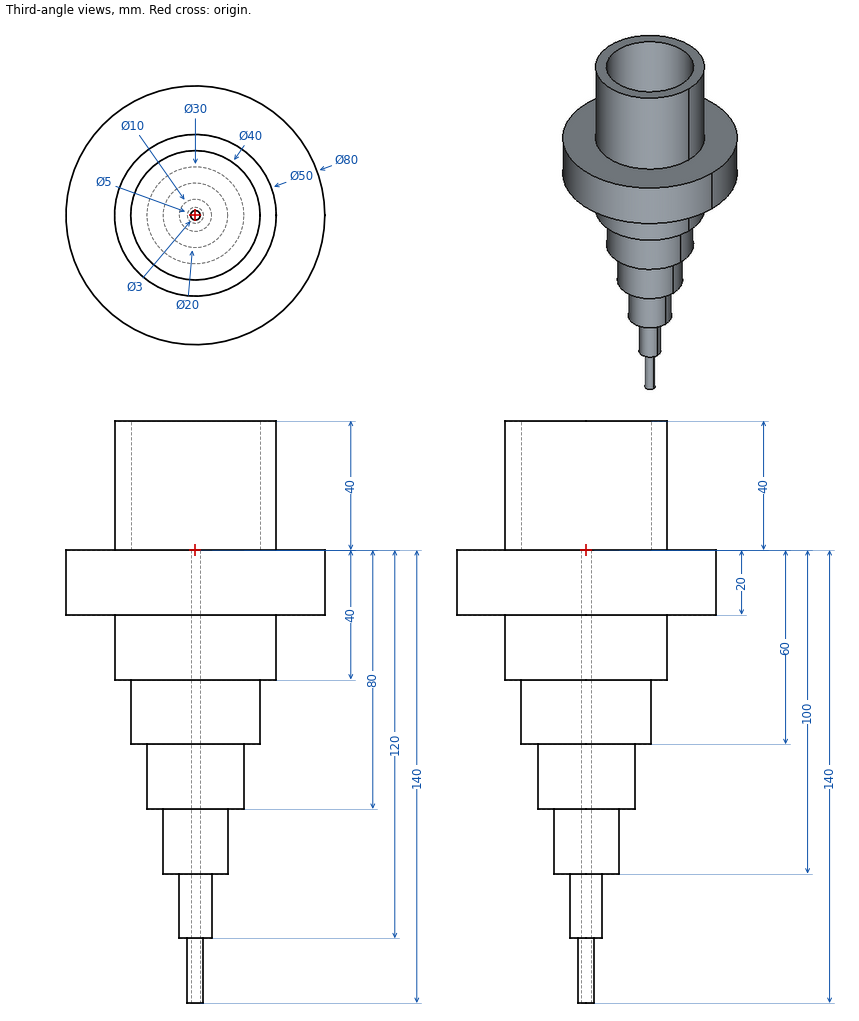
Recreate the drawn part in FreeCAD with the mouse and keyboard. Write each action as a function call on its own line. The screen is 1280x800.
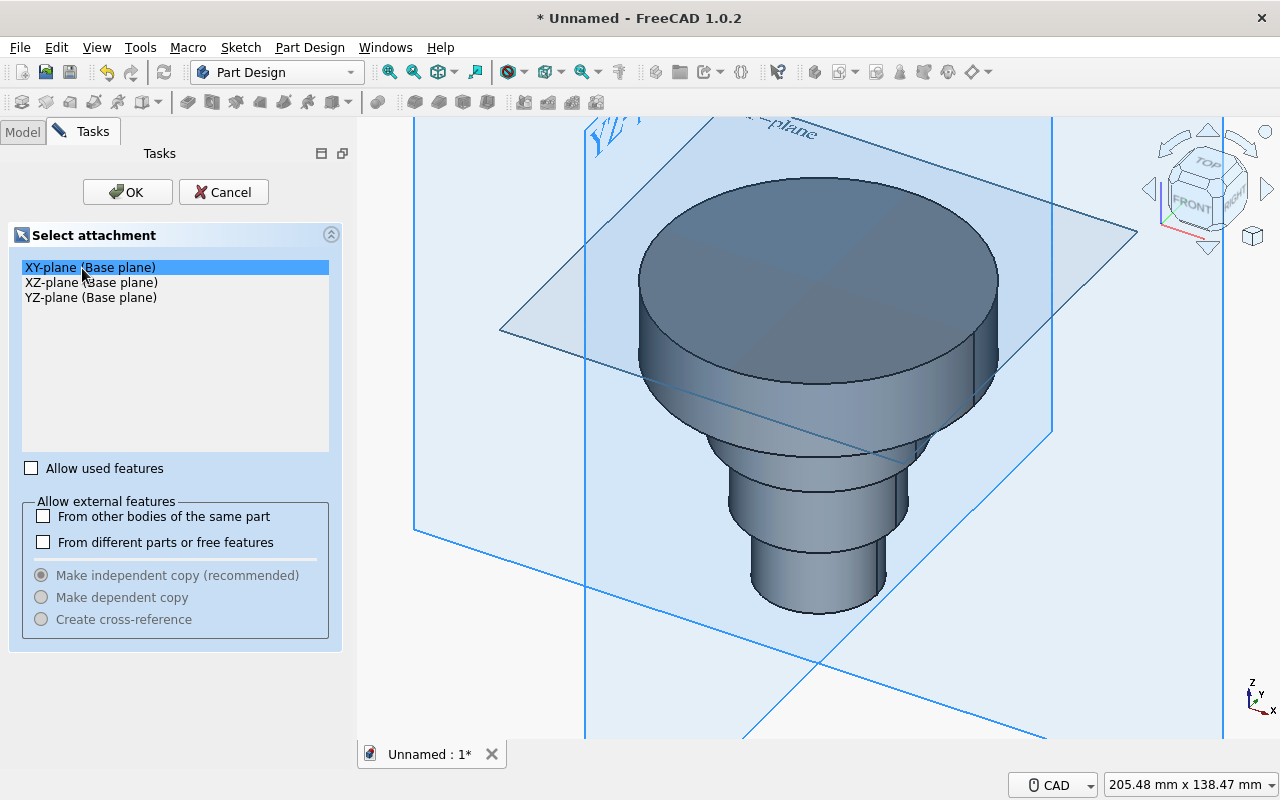
click(128, 192)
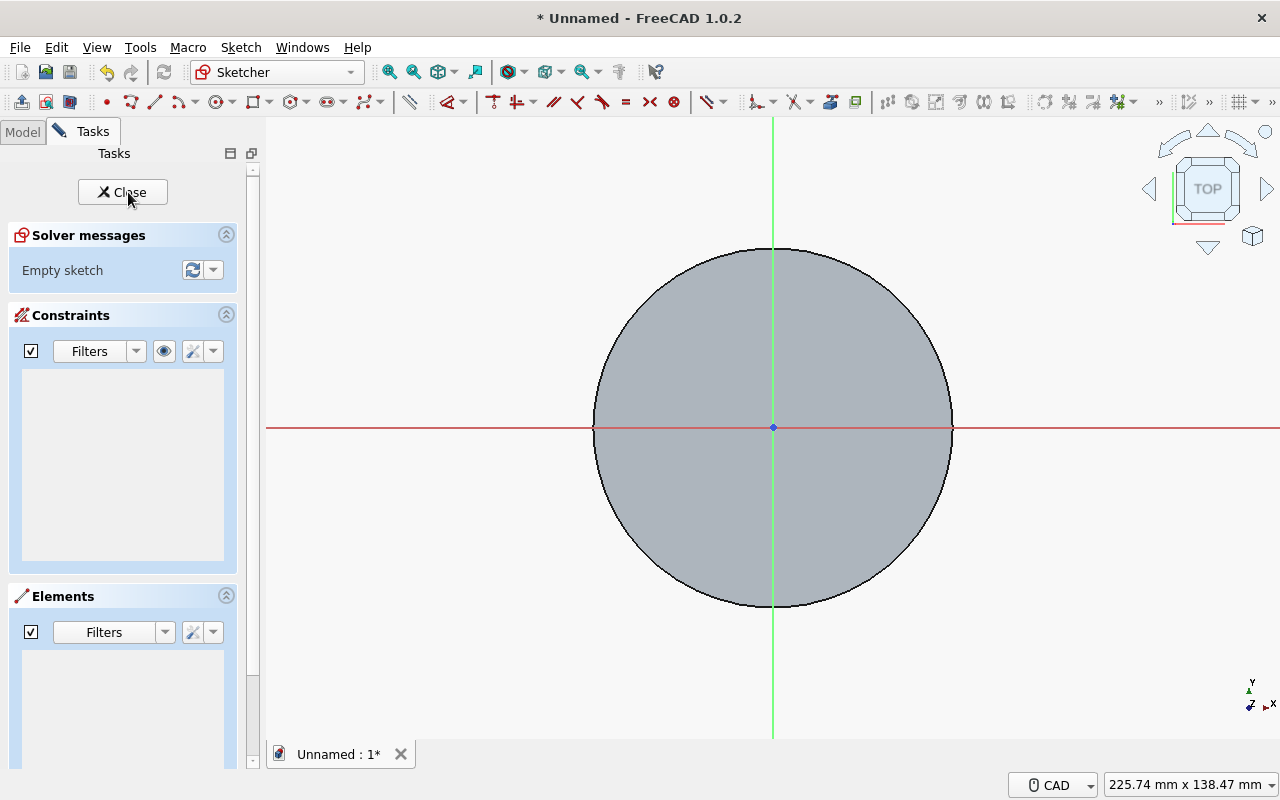
scroll(795, 428, up, 7)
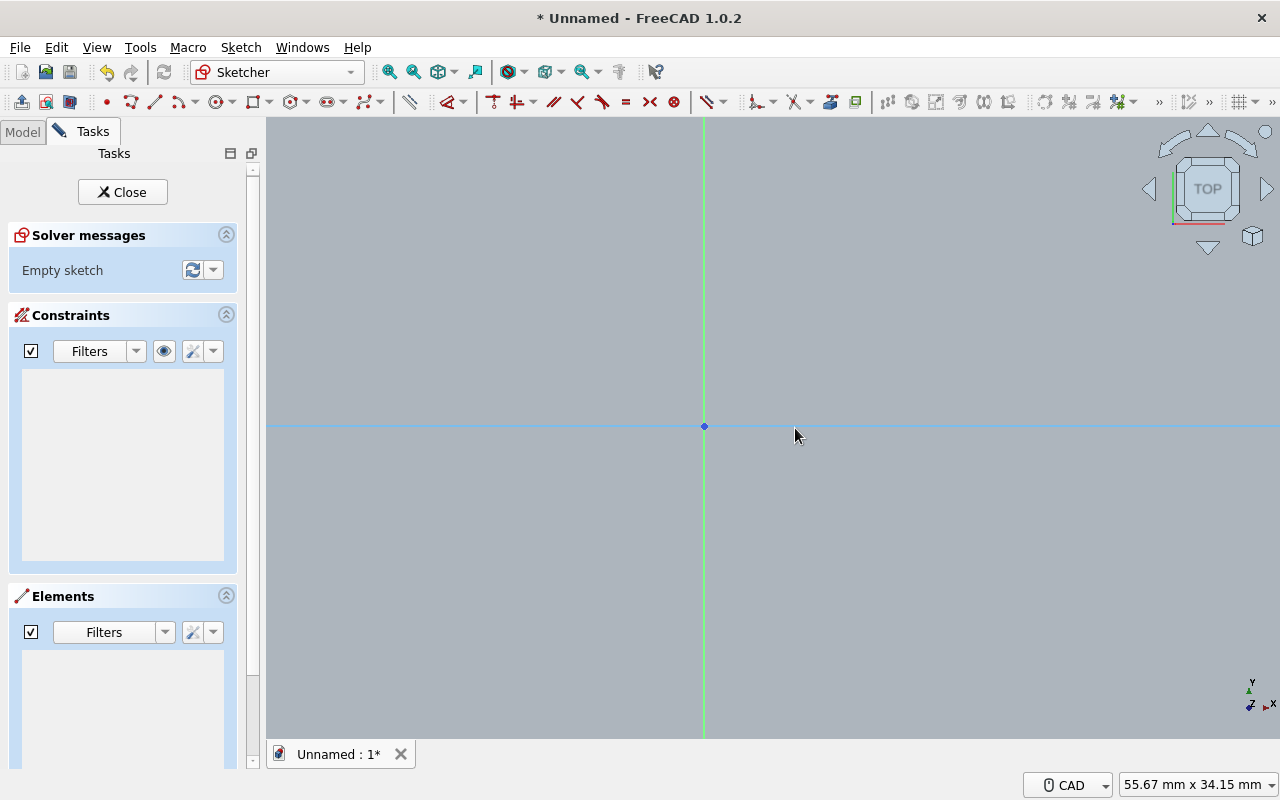
key(g)
key(c)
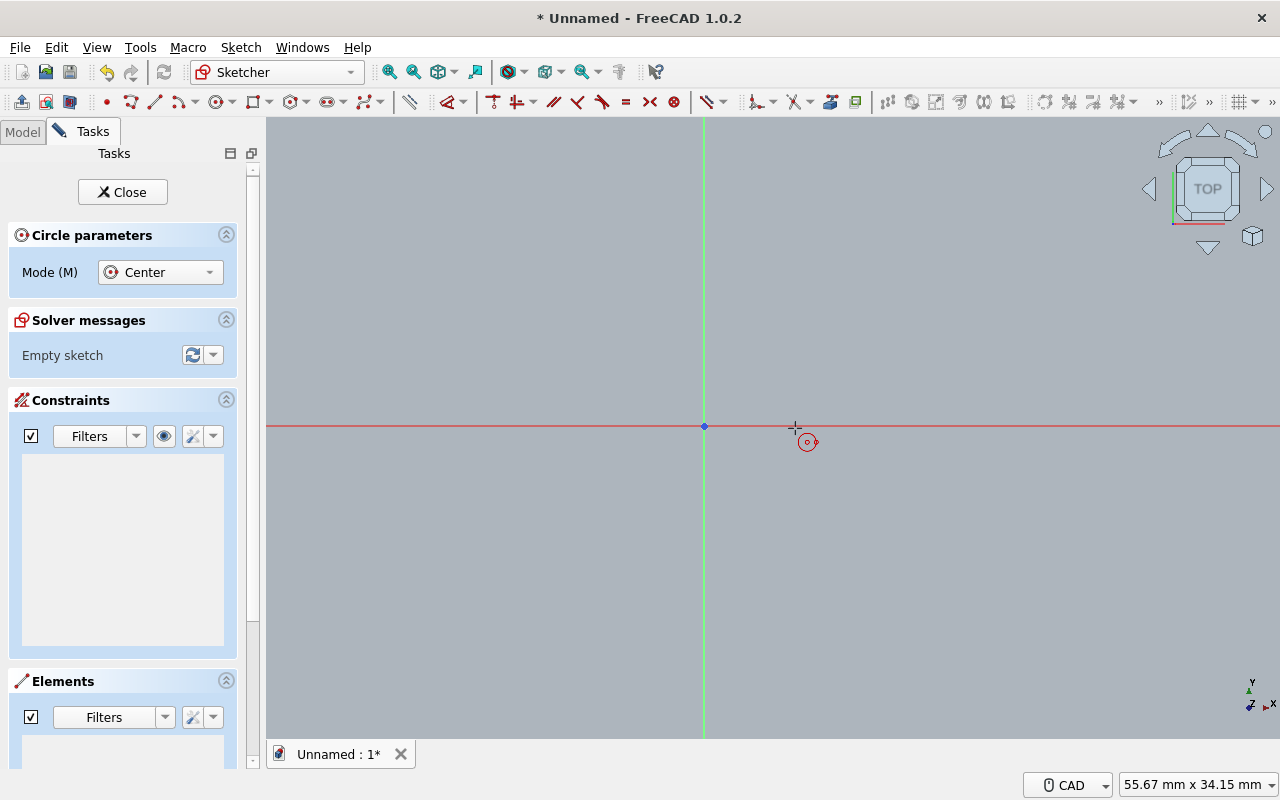
click(704, 426)
move(833, 298)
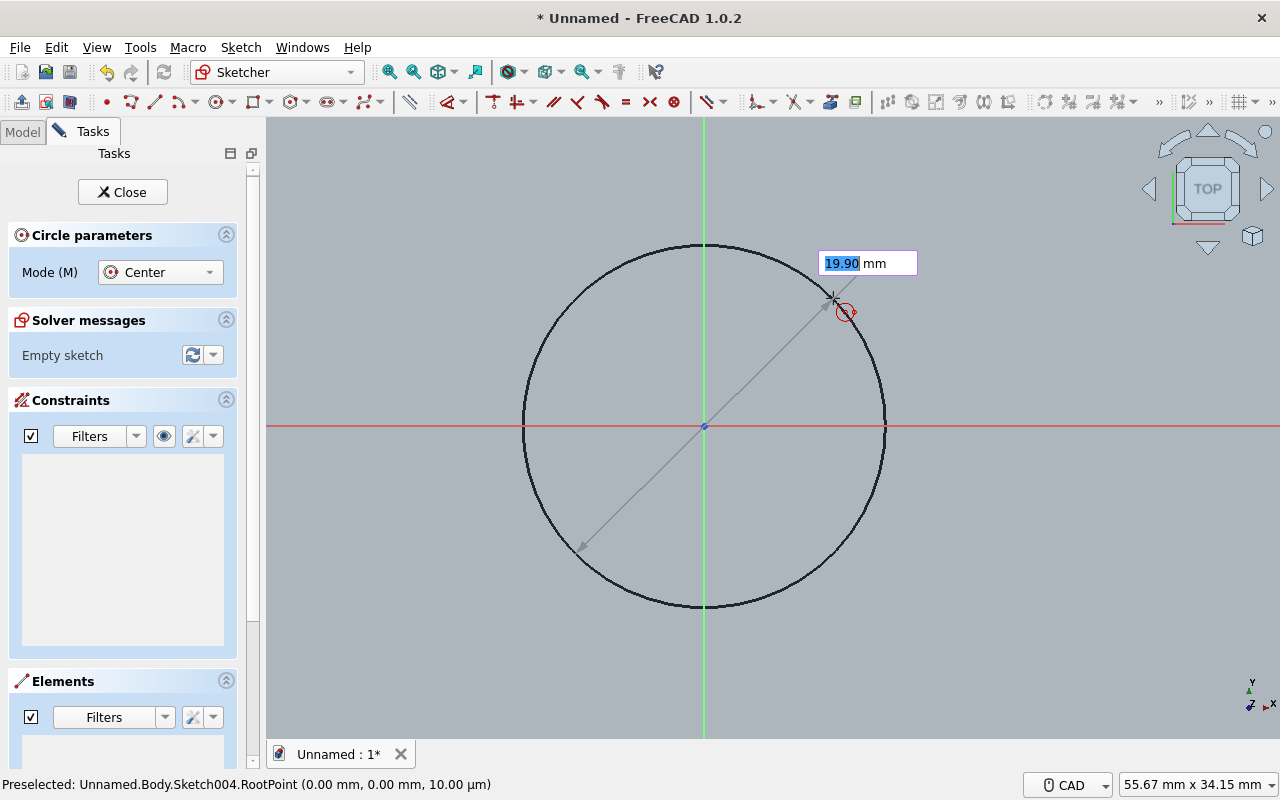
text(20)
key(Return)
key(Escape)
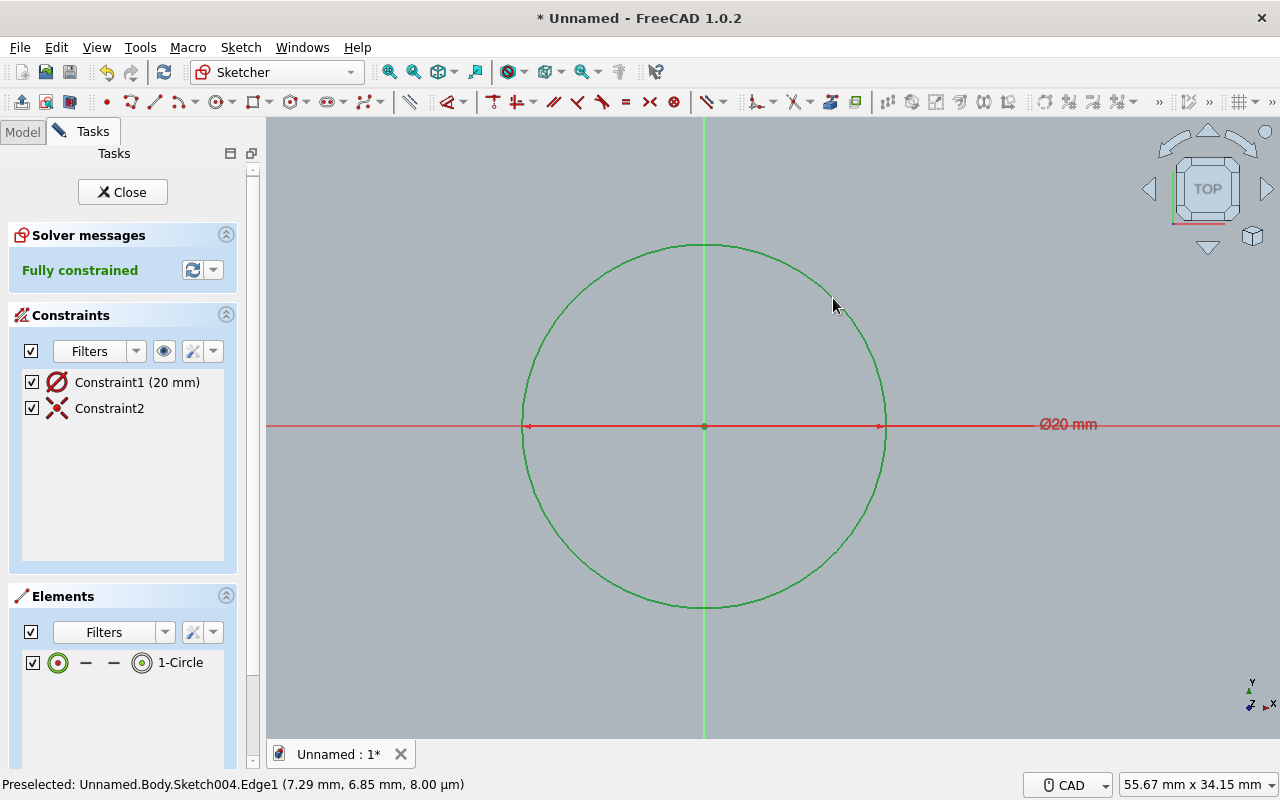
click(123, 192)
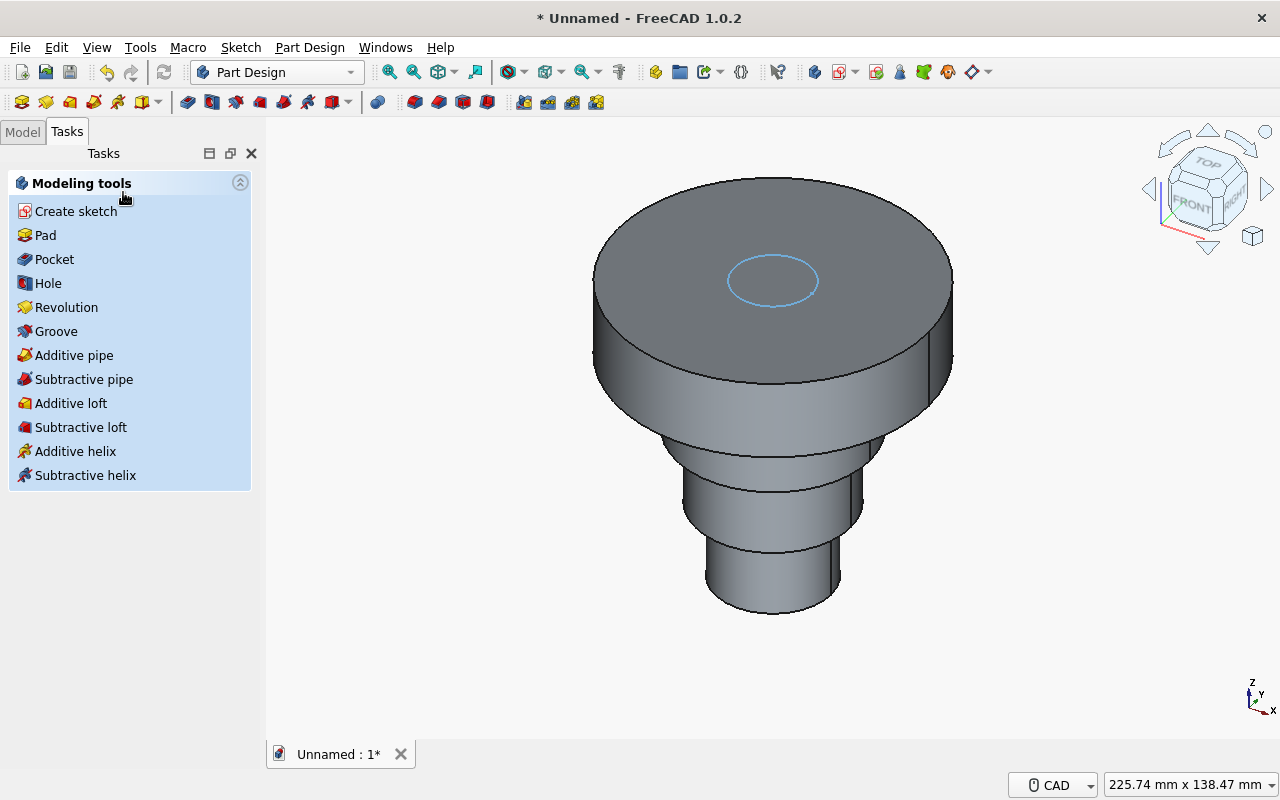
click(22, 102)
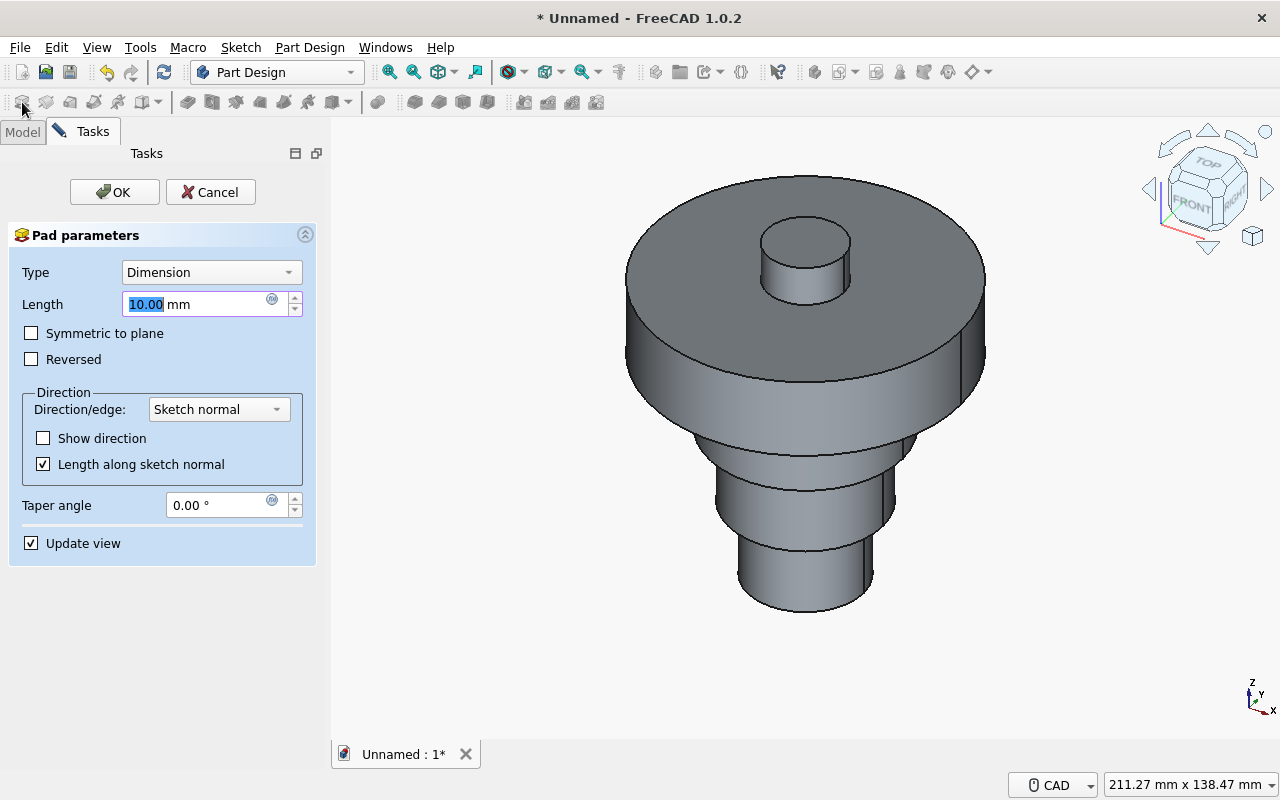
text(100)
key(Tab)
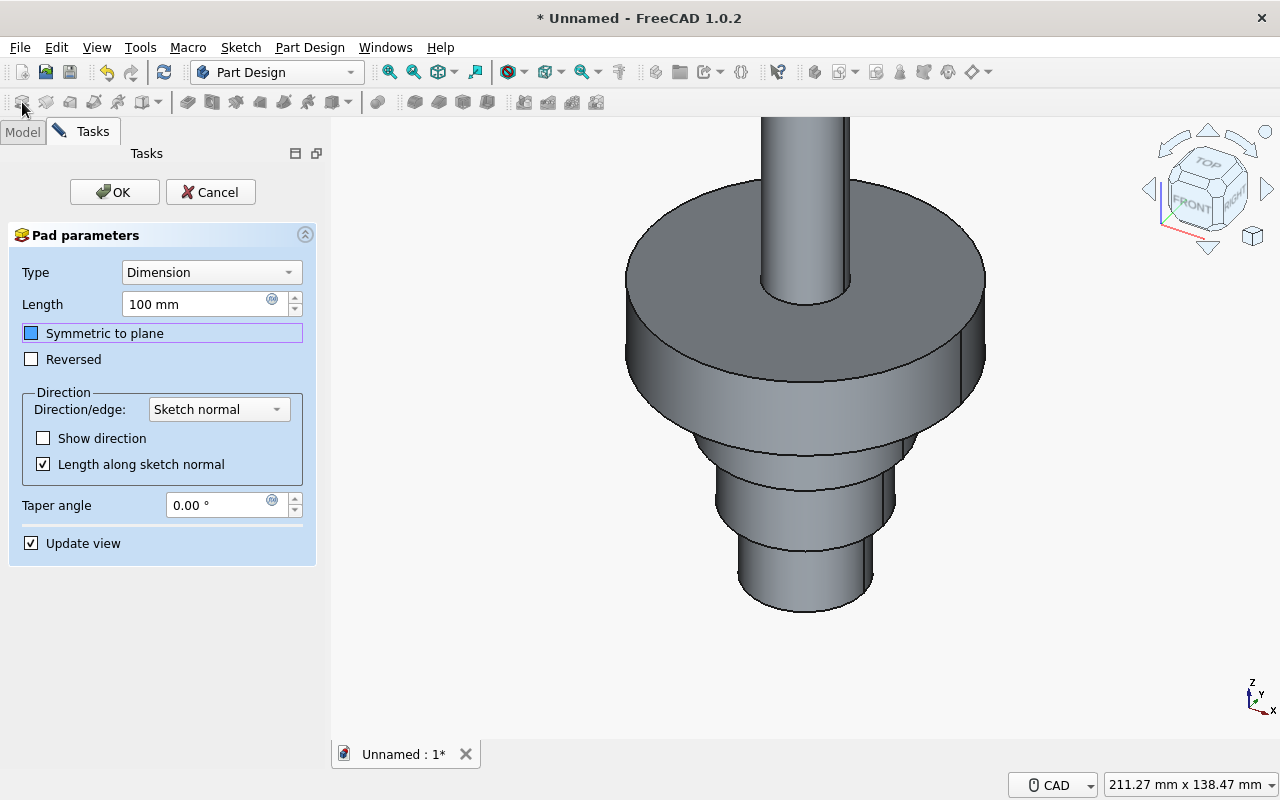
click(30, 359)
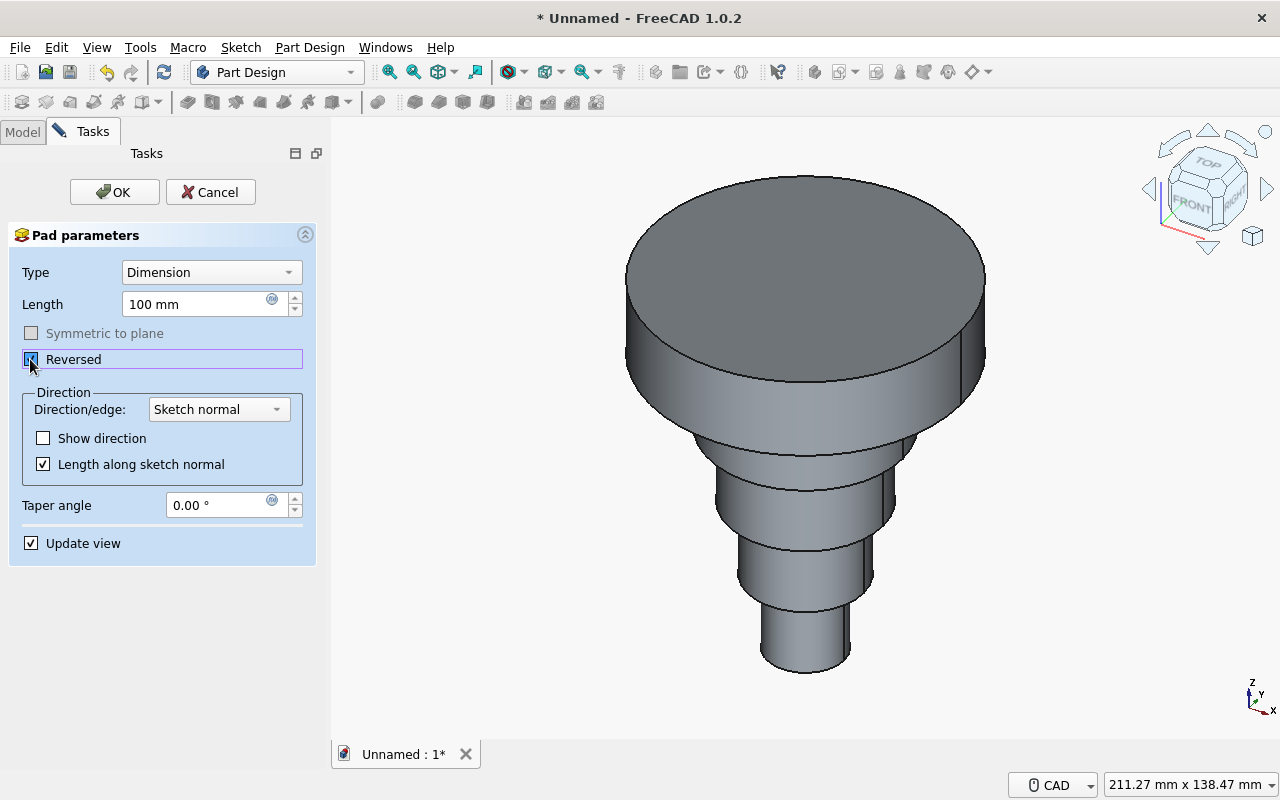
click(115, 192)